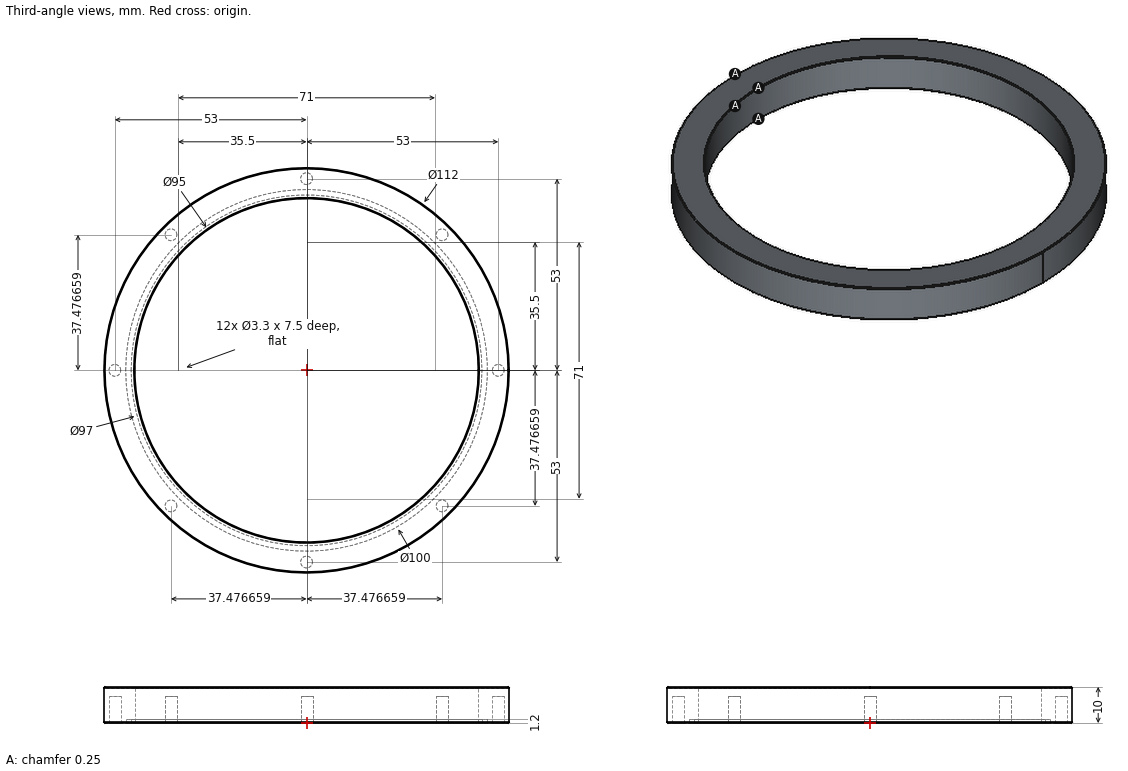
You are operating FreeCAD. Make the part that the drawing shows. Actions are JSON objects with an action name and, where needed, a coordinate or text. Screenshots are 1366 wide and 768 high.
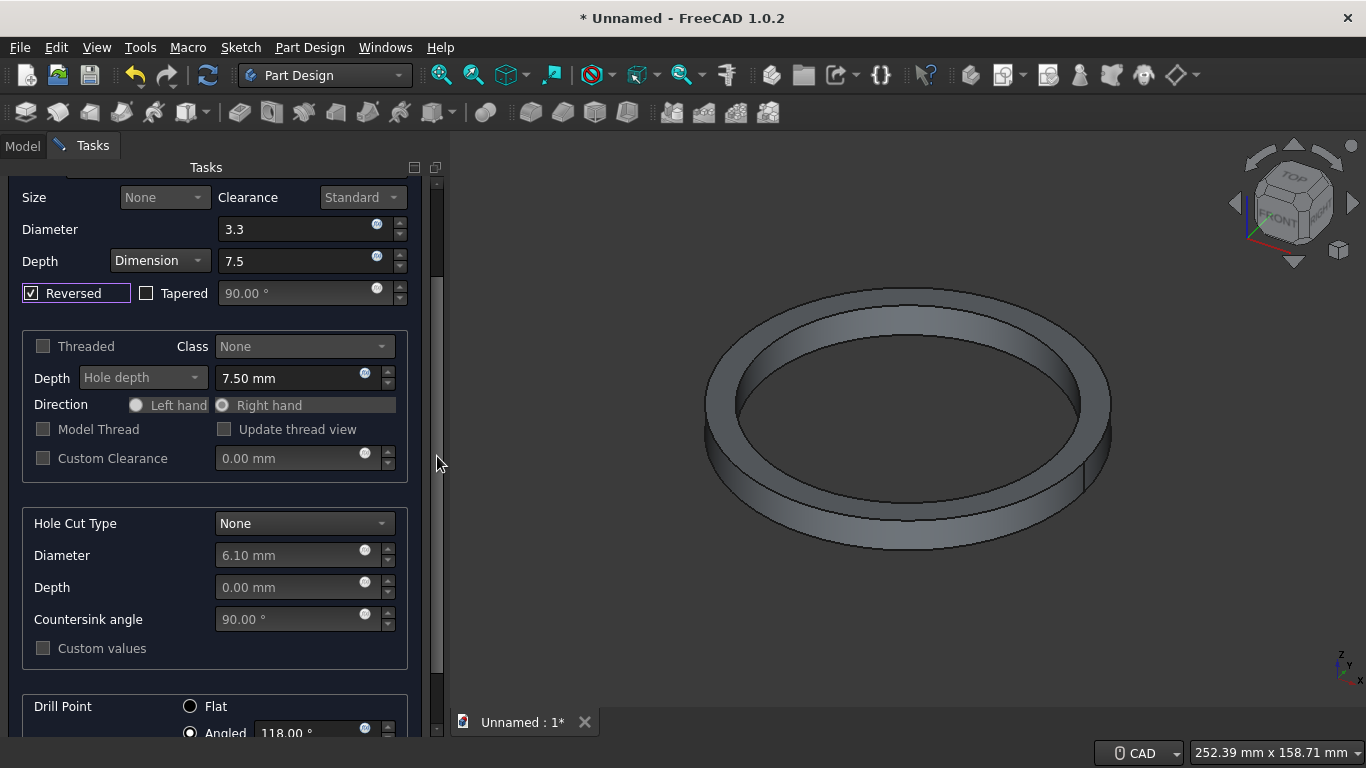
{"action": "left_click", "coordinate": [191, 646]}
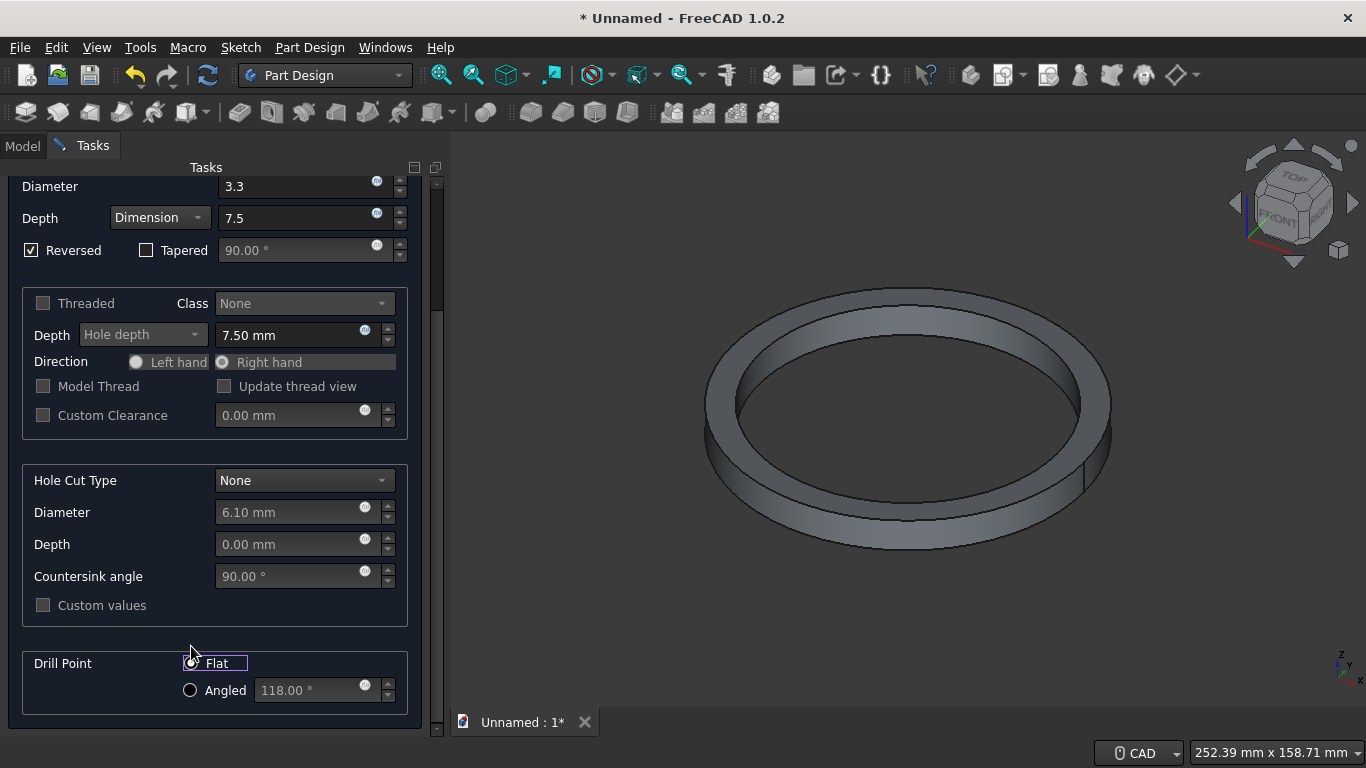
{"action": "scroll", "coordinate": [437, 456], "scroll_direction": "up", "scroll_amount": 4}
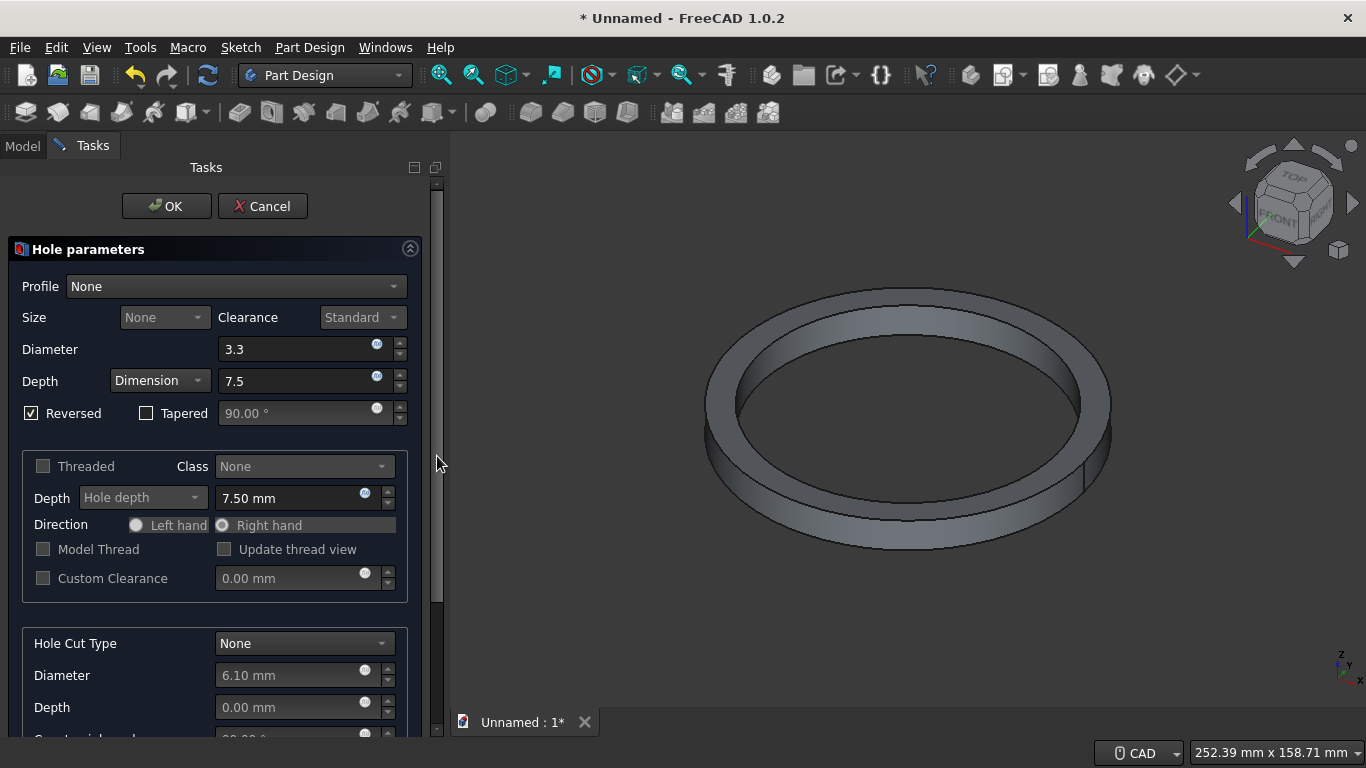
{"action": "left_click", "coordinate": [167, 206]}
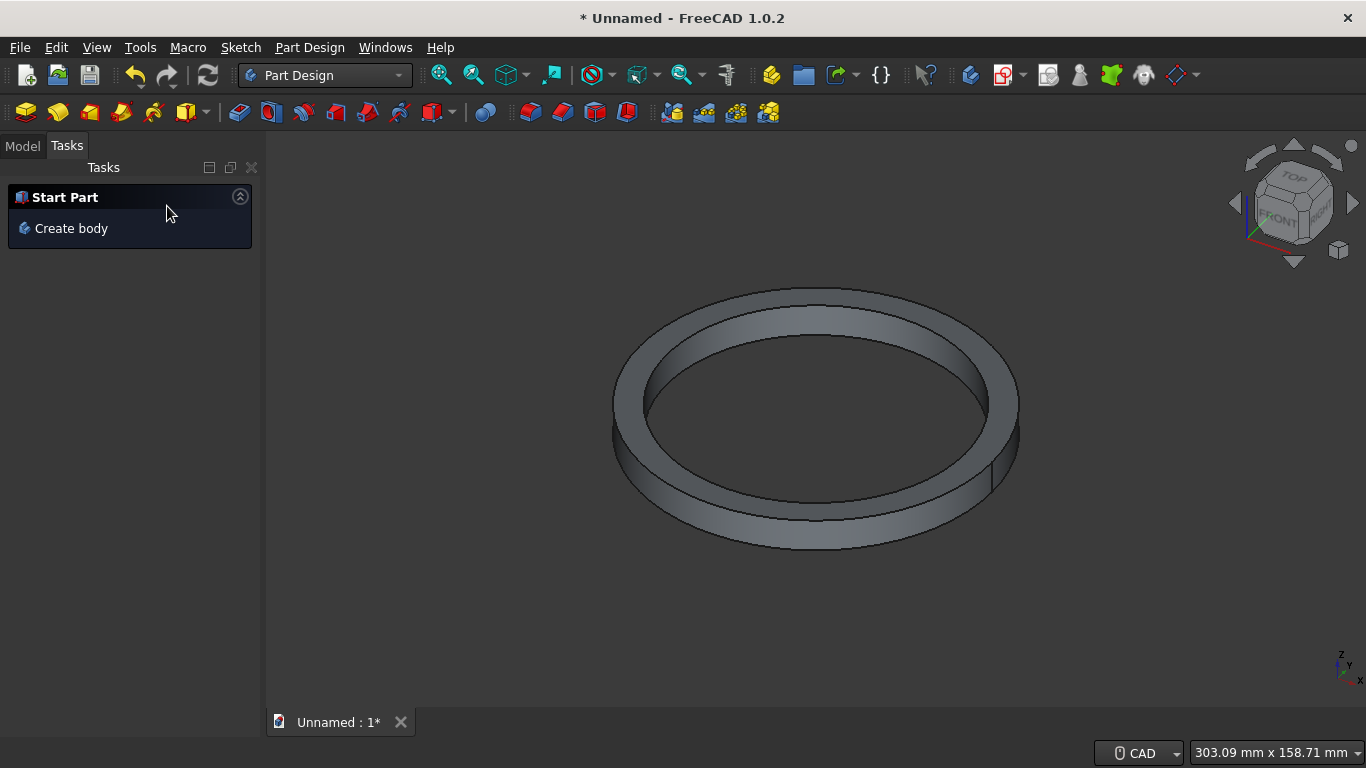
{"action": "left_click", "coordinate": [614, 415]}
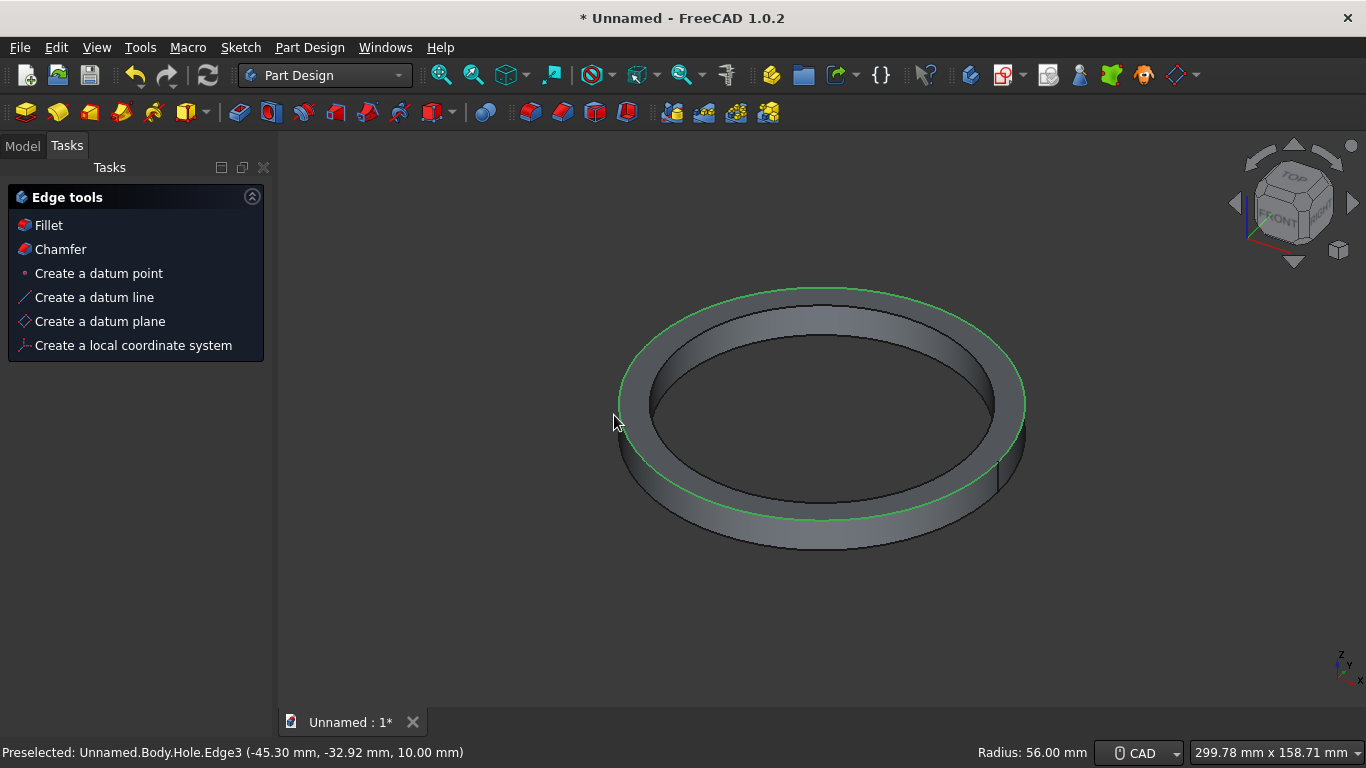
{"action": "left_click", "coordinate": [673, 354], "text": "ctrl"}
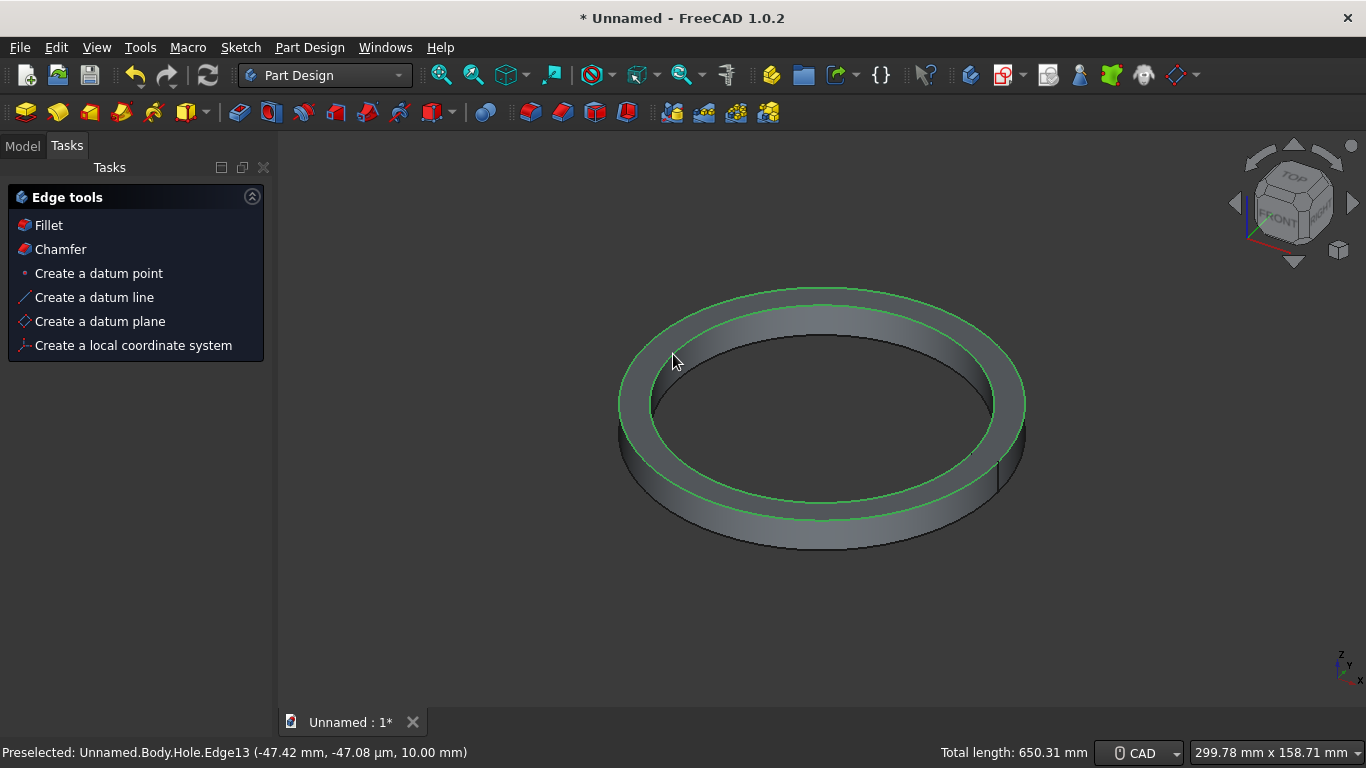
{"action": "key", "text": "0"}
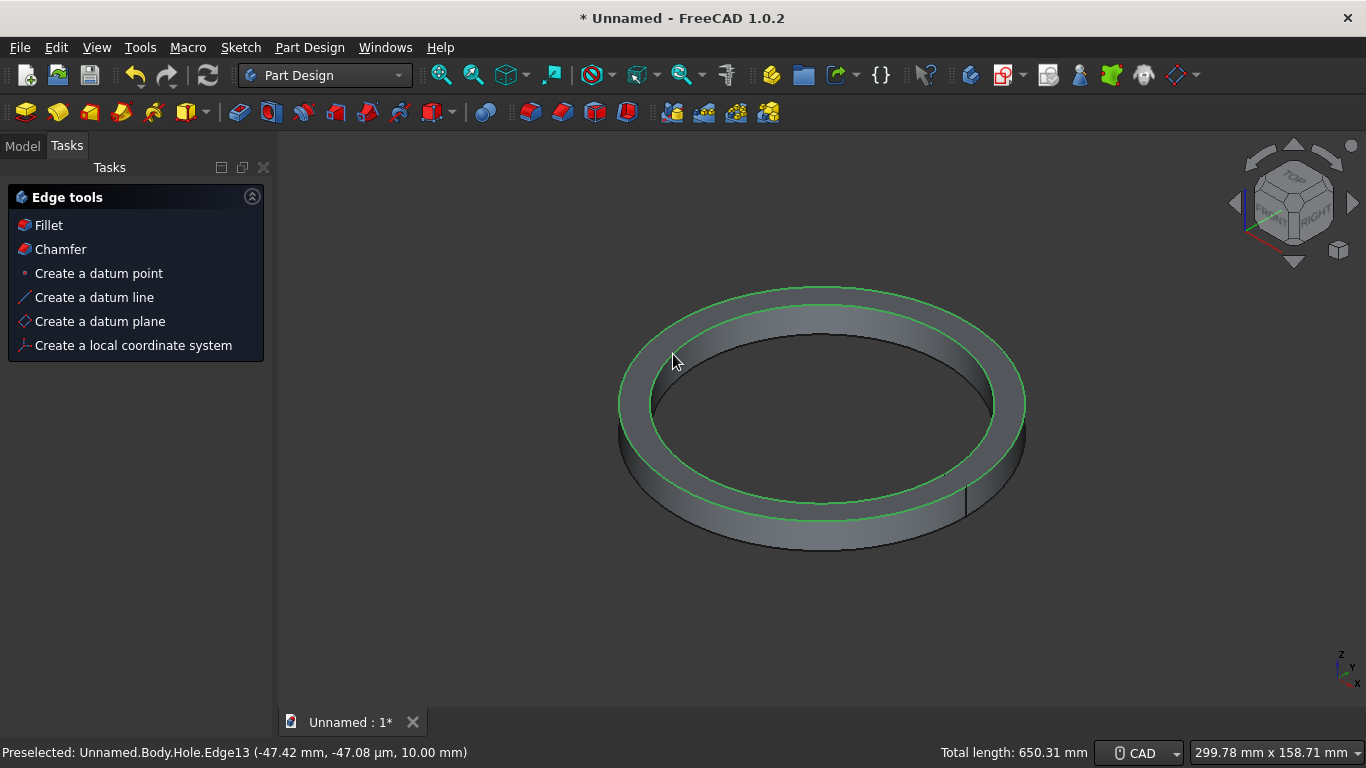
{"action": "key", "text": "2"}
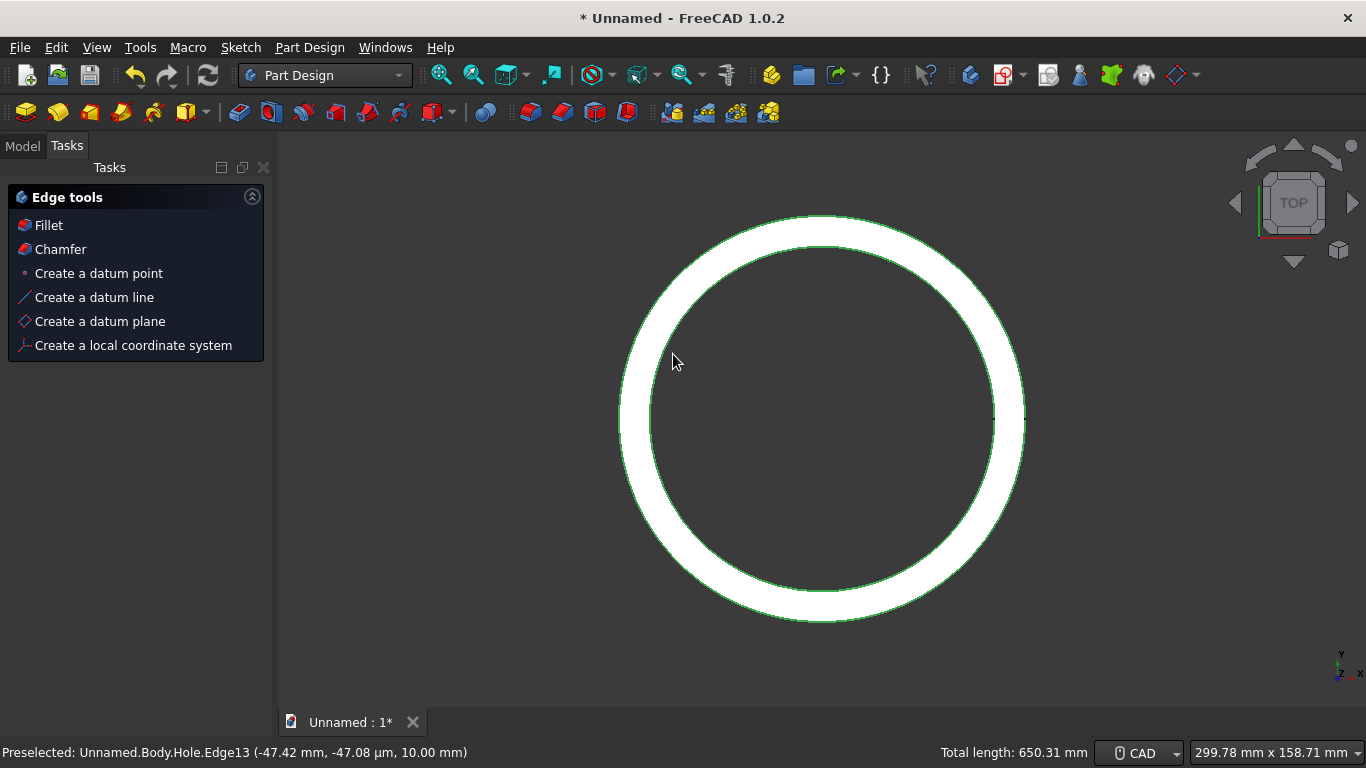
{"action": "key", "text": "1"}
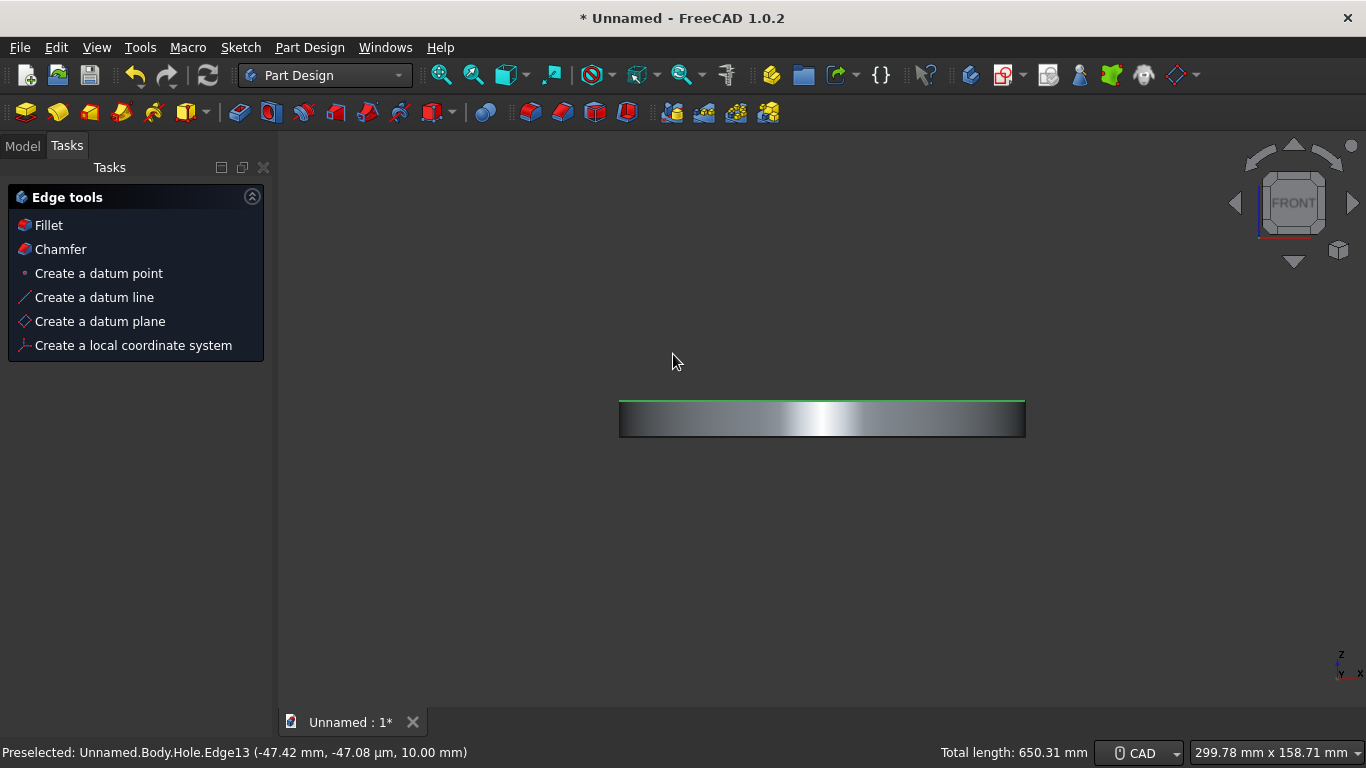
{"action": "left_click", "coordinate": [442, 76]}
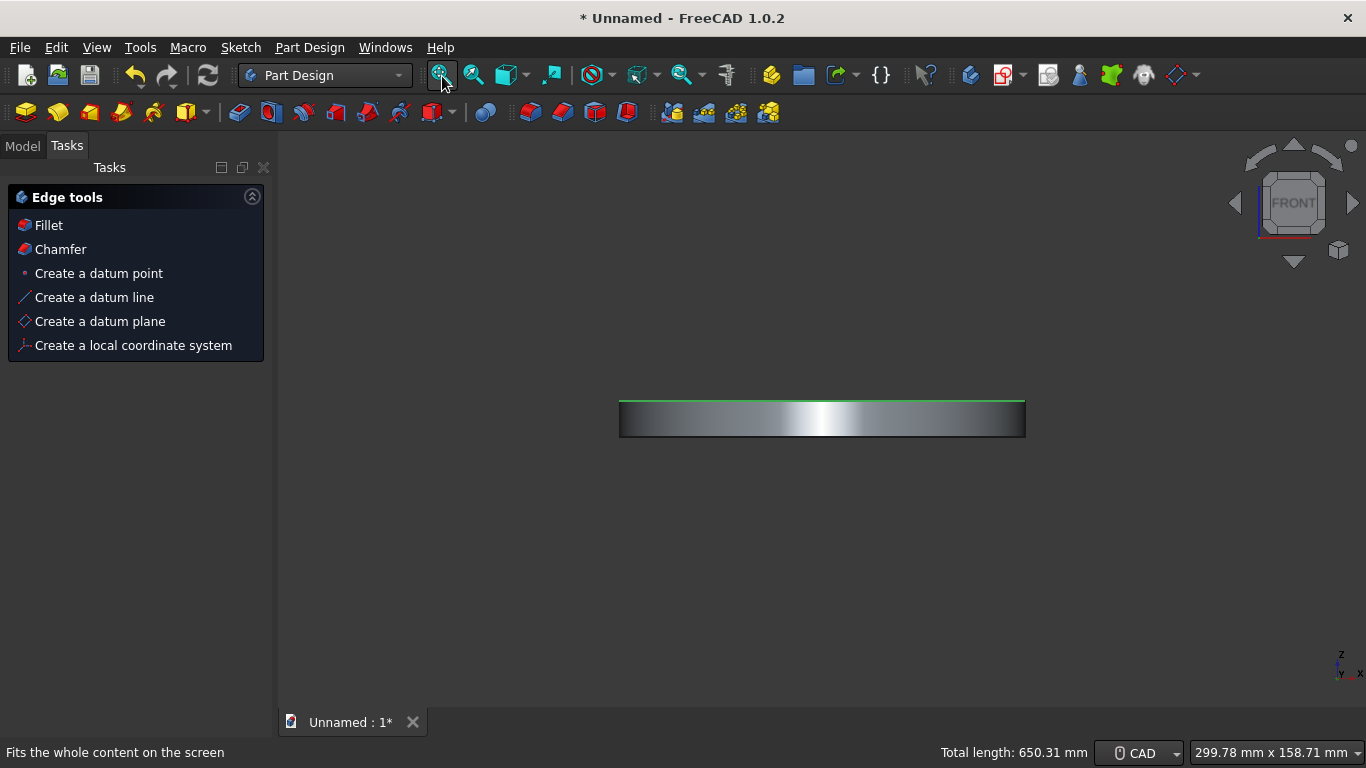
{"action": "left_click", "coordinate": [658, 436], "text": "ctrl"}